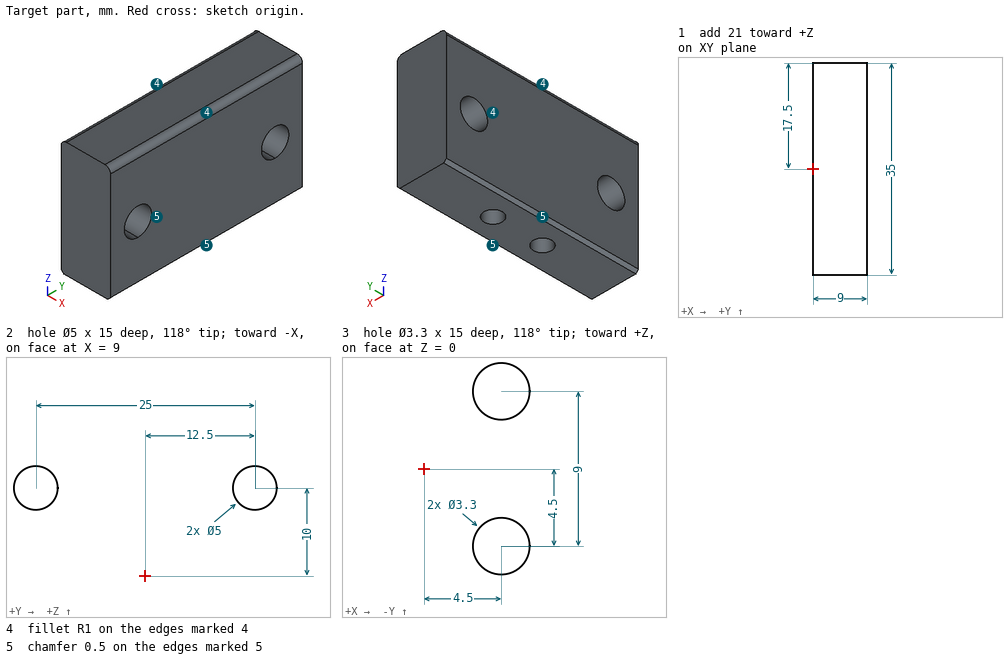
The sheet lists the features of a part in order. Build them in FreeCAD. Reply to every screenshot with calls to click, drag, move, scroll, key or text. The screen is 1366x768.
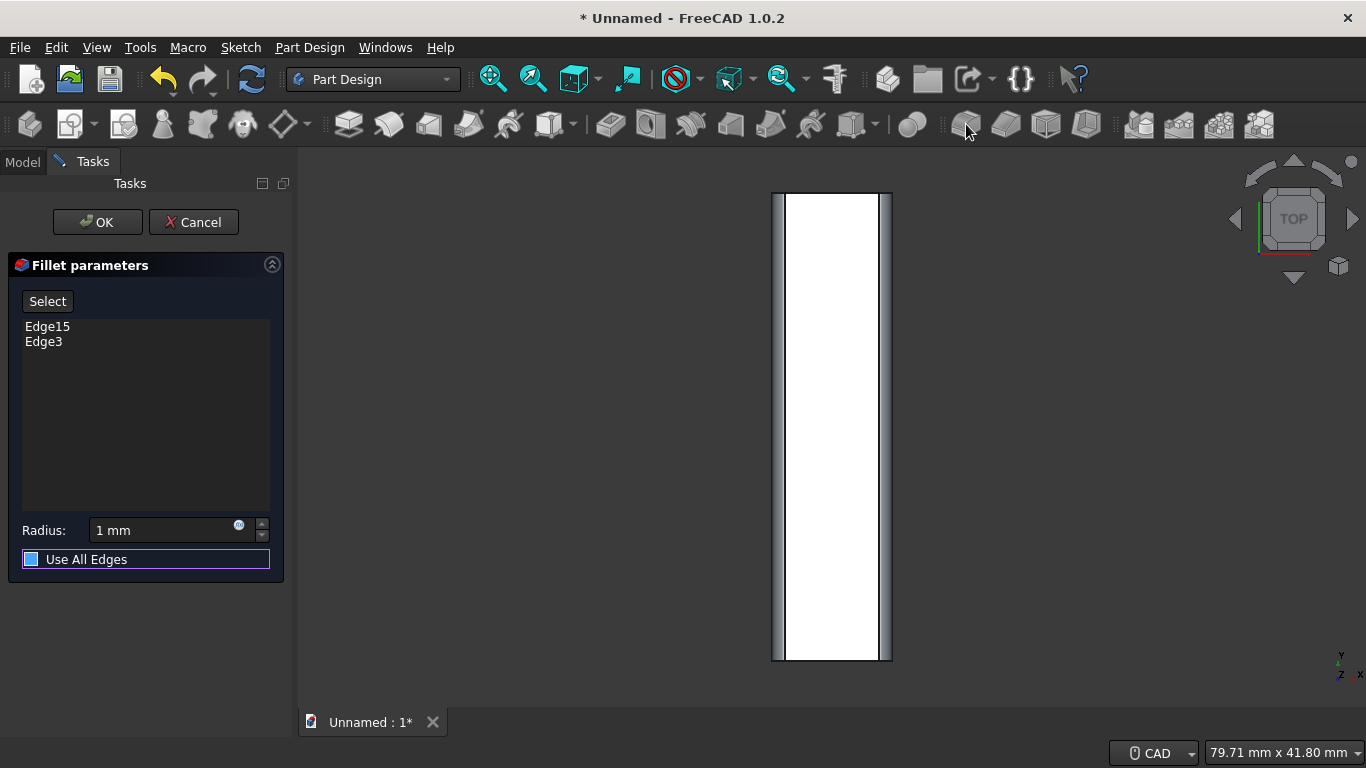
click(98, 222)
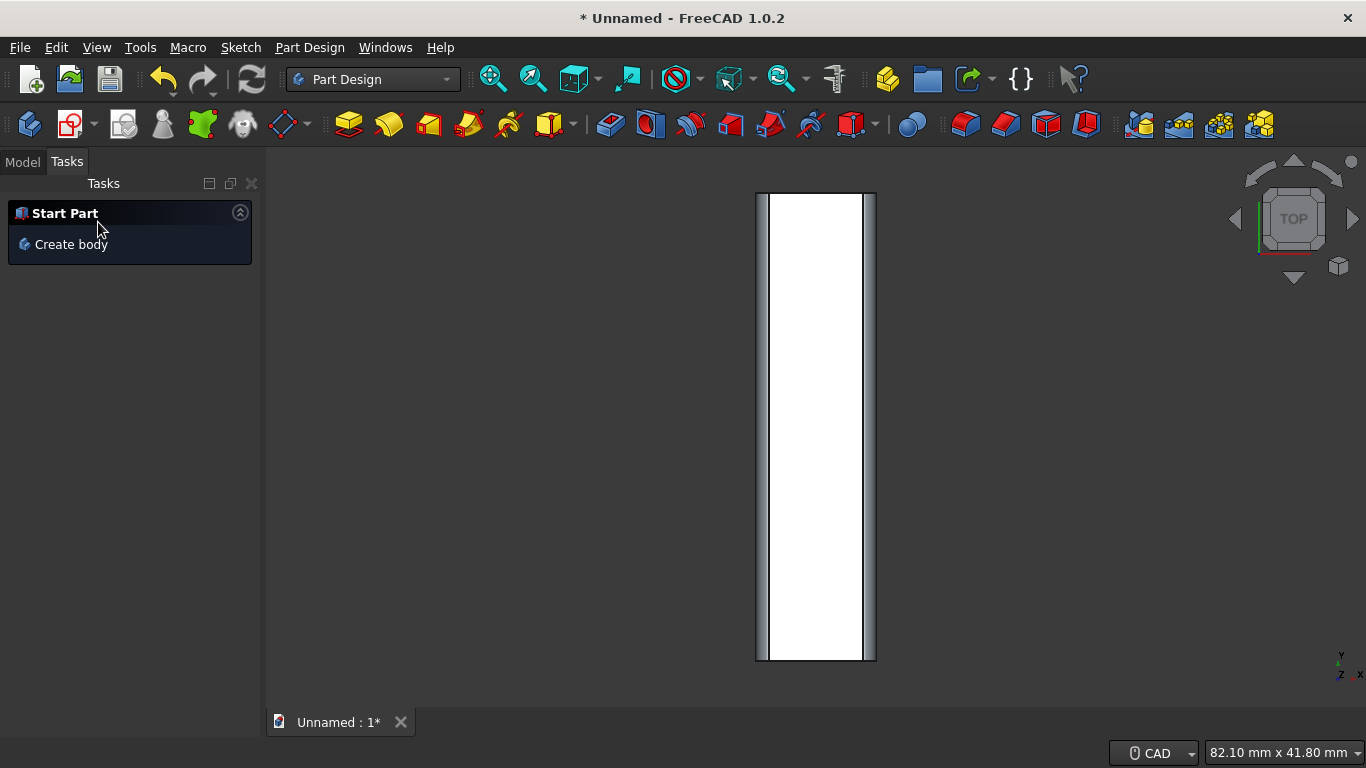
key(0)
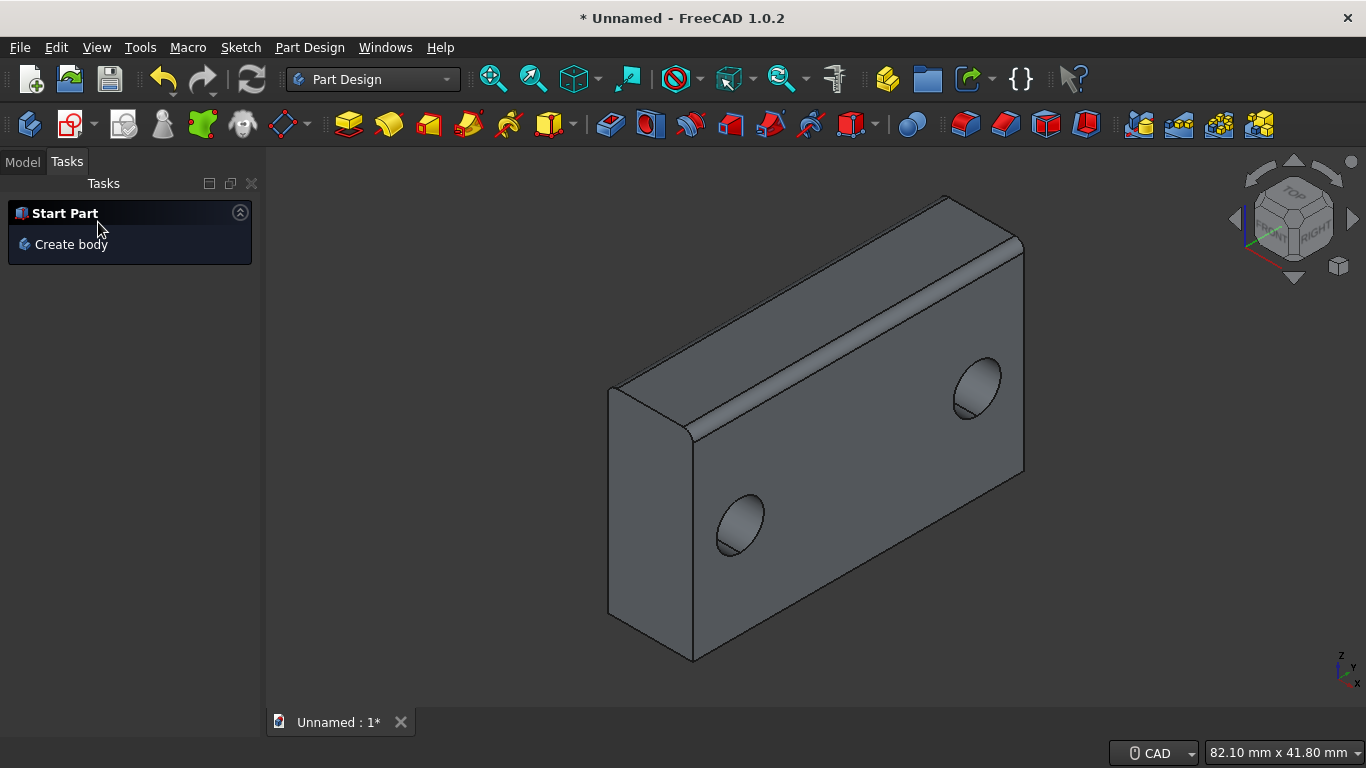
key(2)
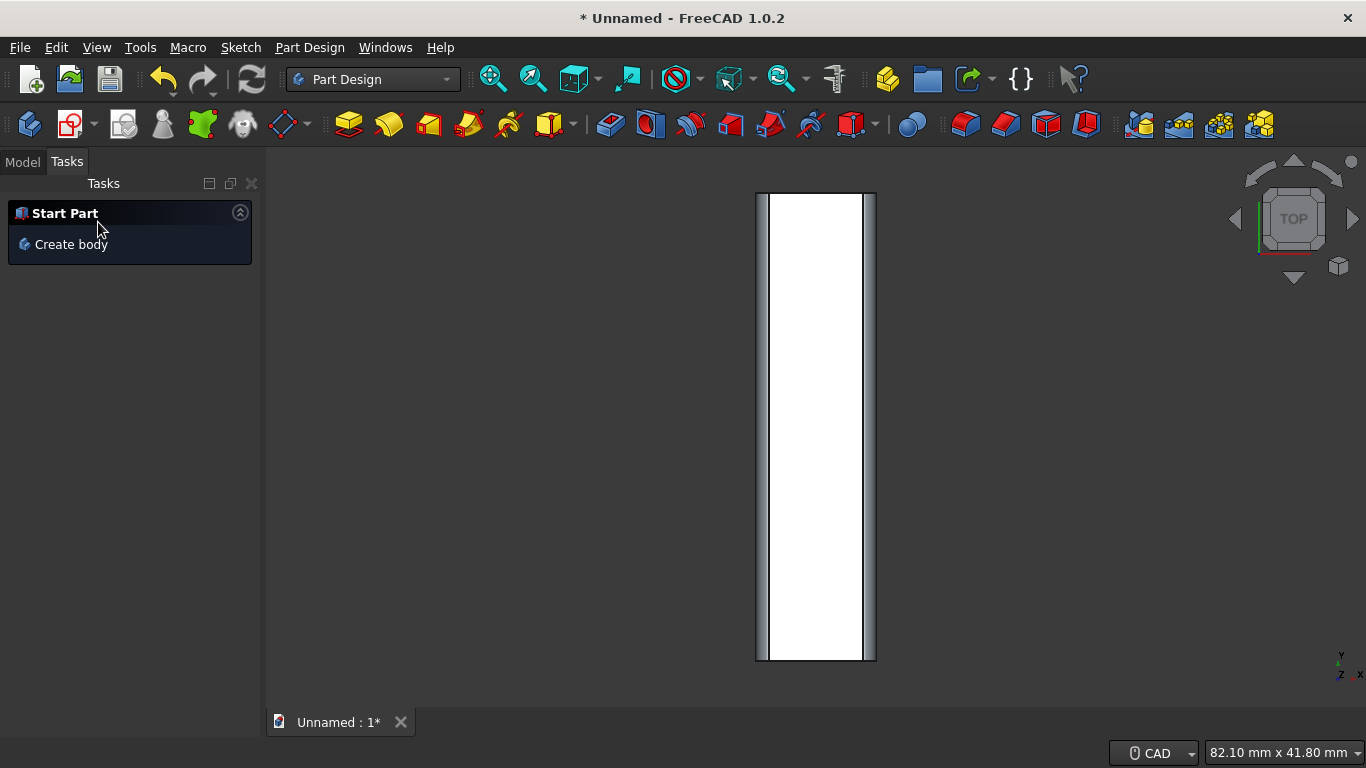
key(1)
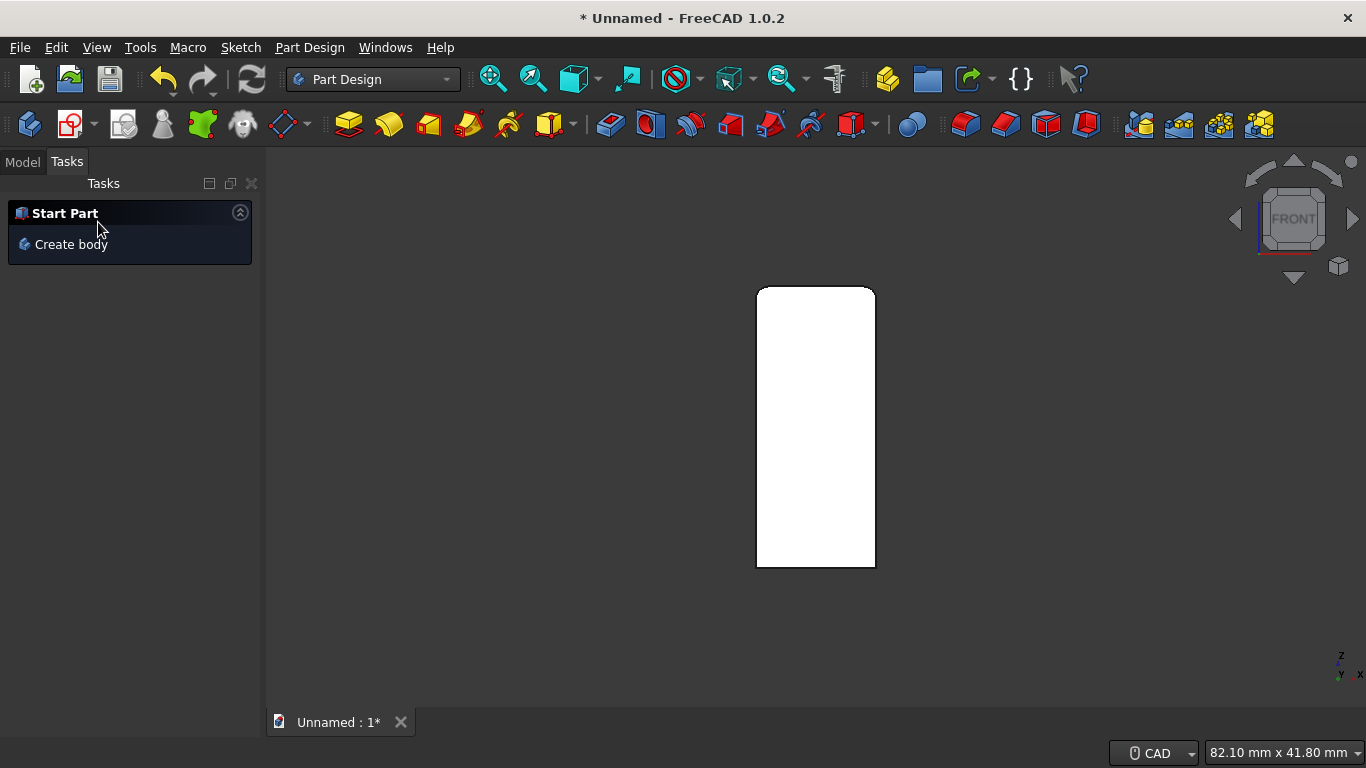
key(3)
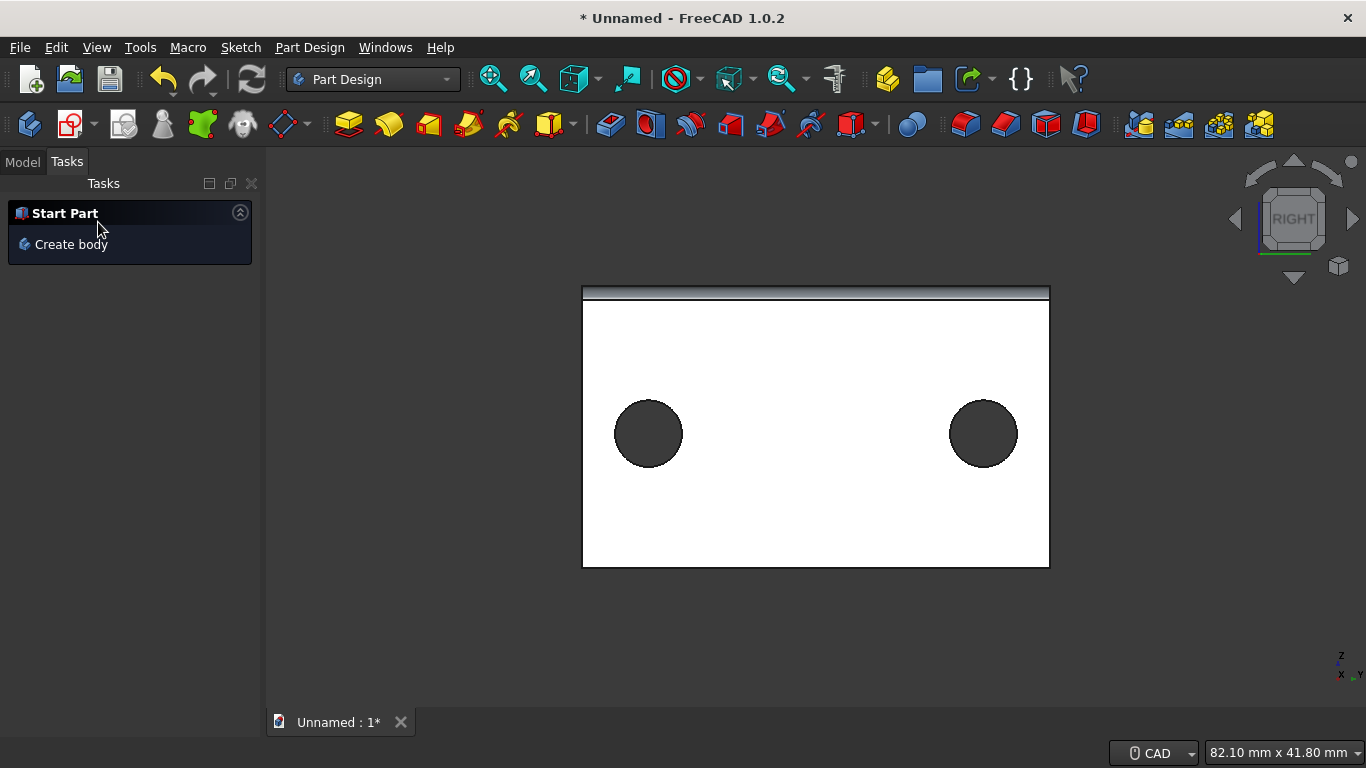
click(816, 567)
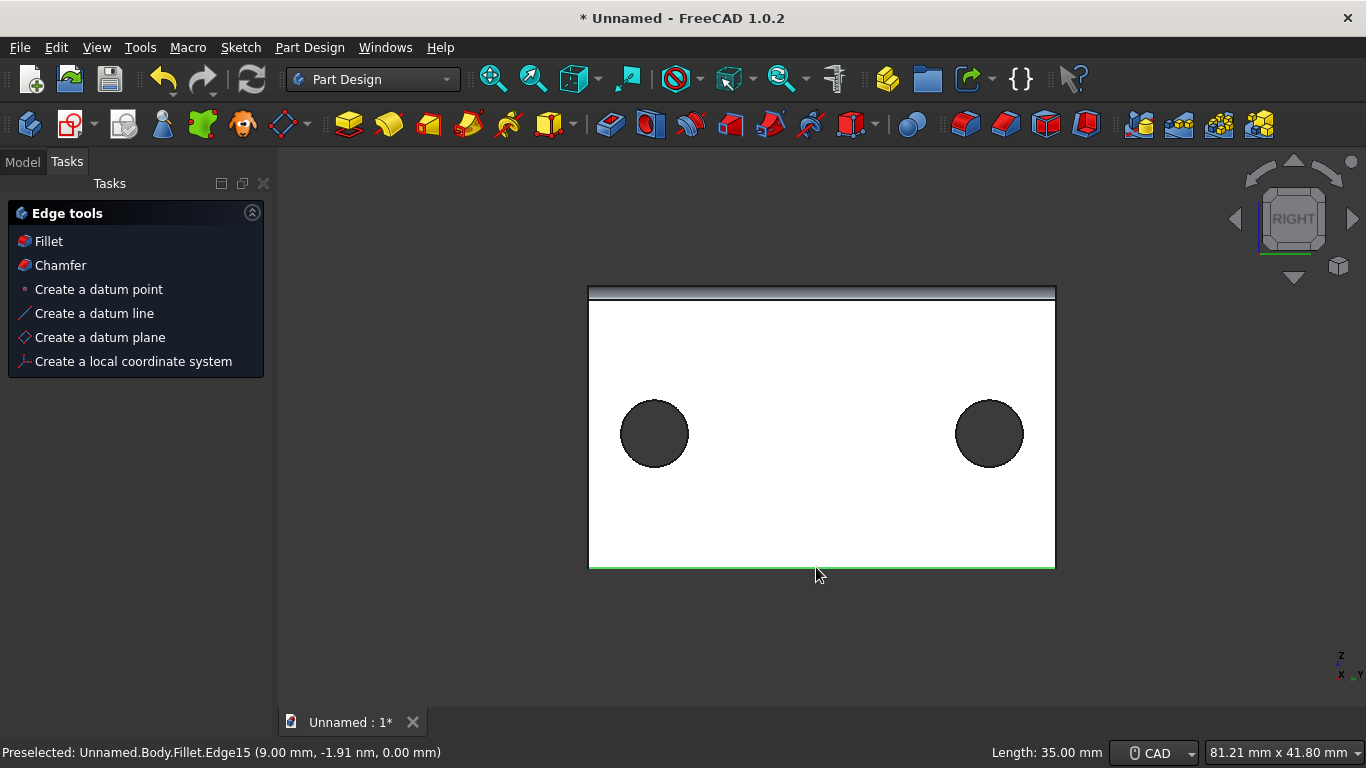
key(5)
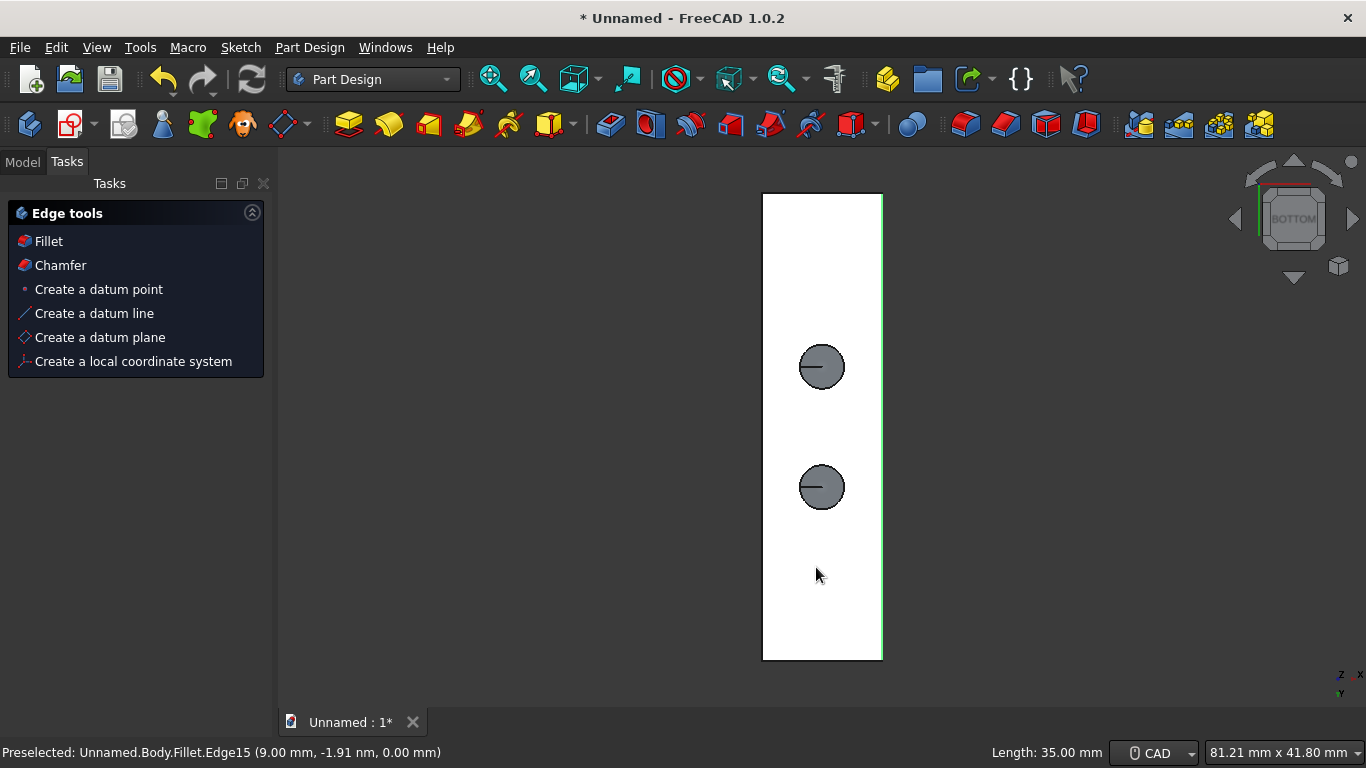
click(762, 426, ctrl)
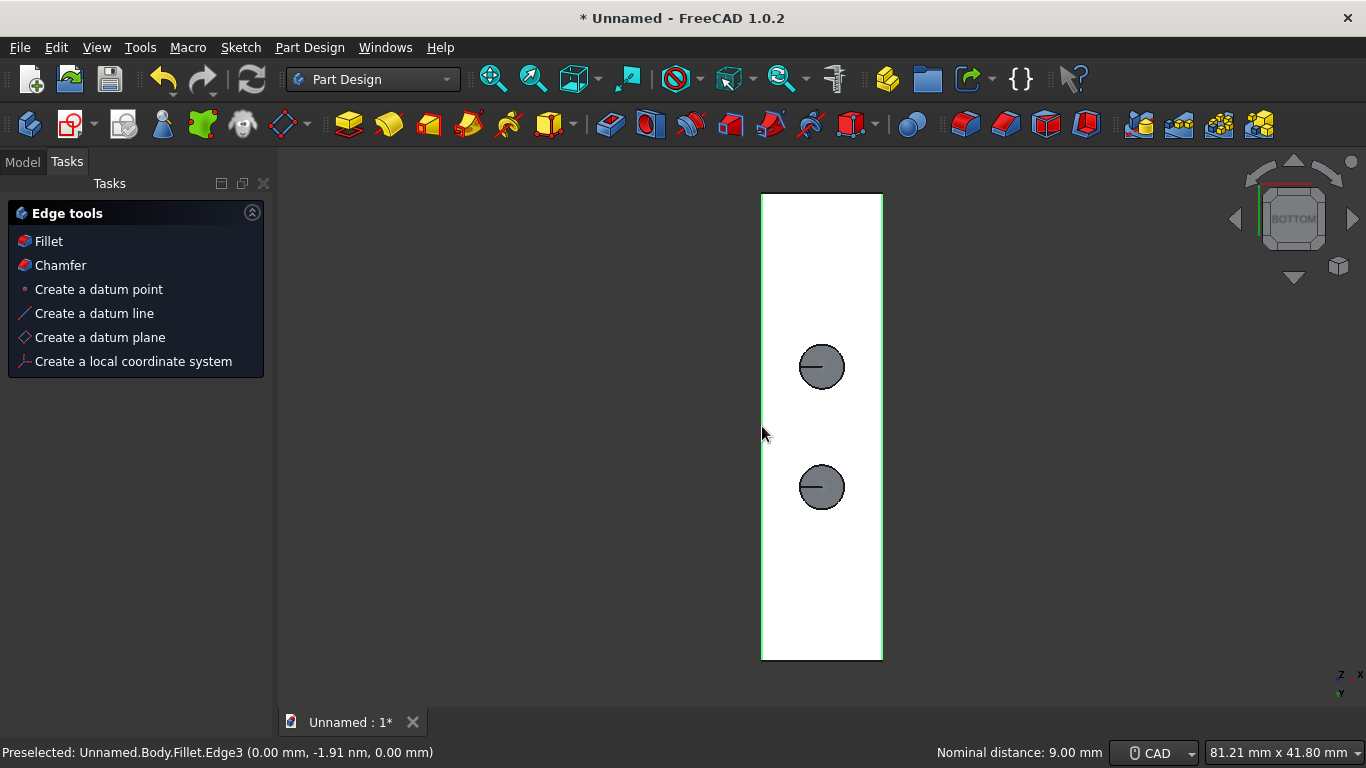
click(1006, 124)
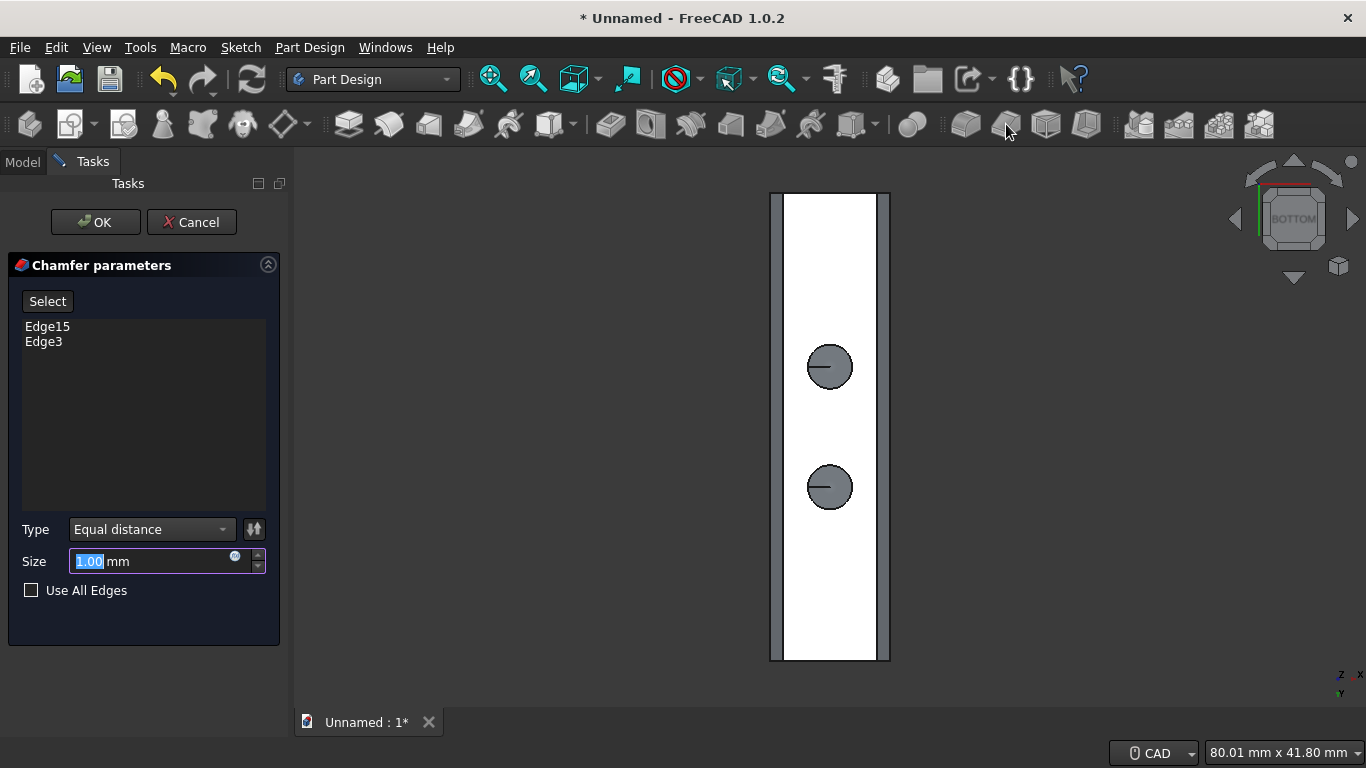
text(0.5)
key(Tab)